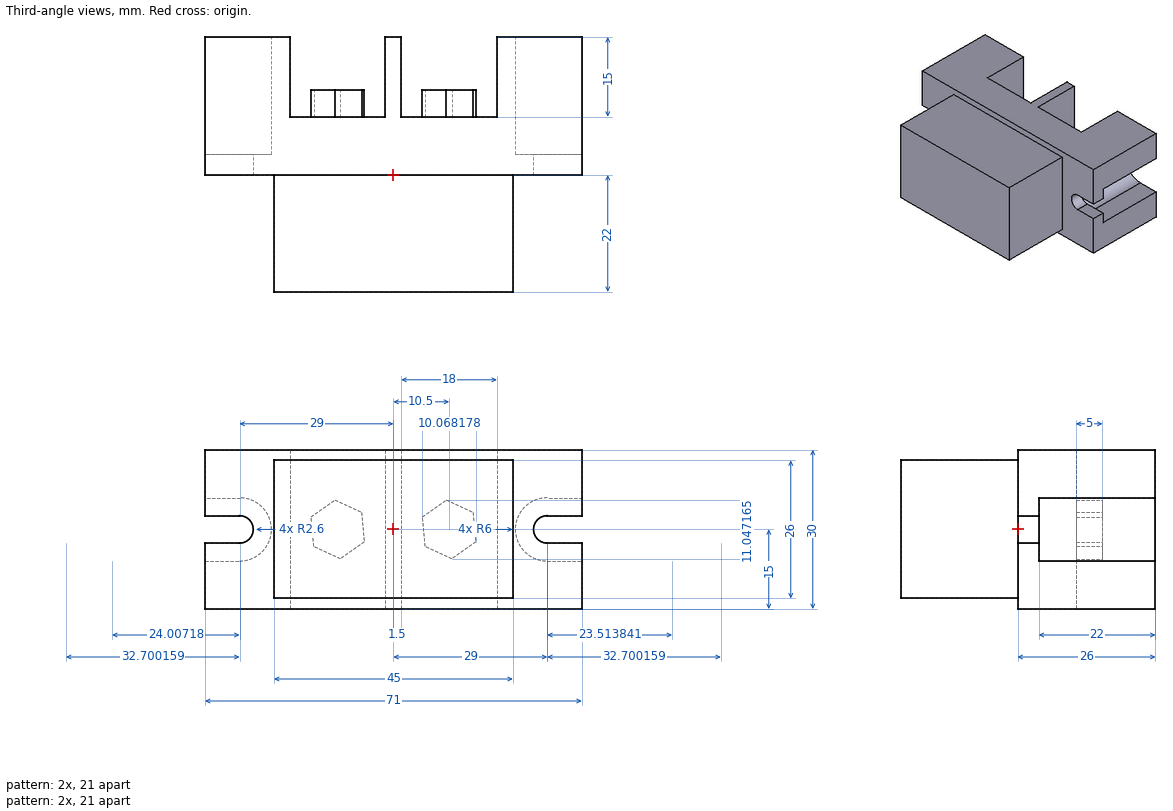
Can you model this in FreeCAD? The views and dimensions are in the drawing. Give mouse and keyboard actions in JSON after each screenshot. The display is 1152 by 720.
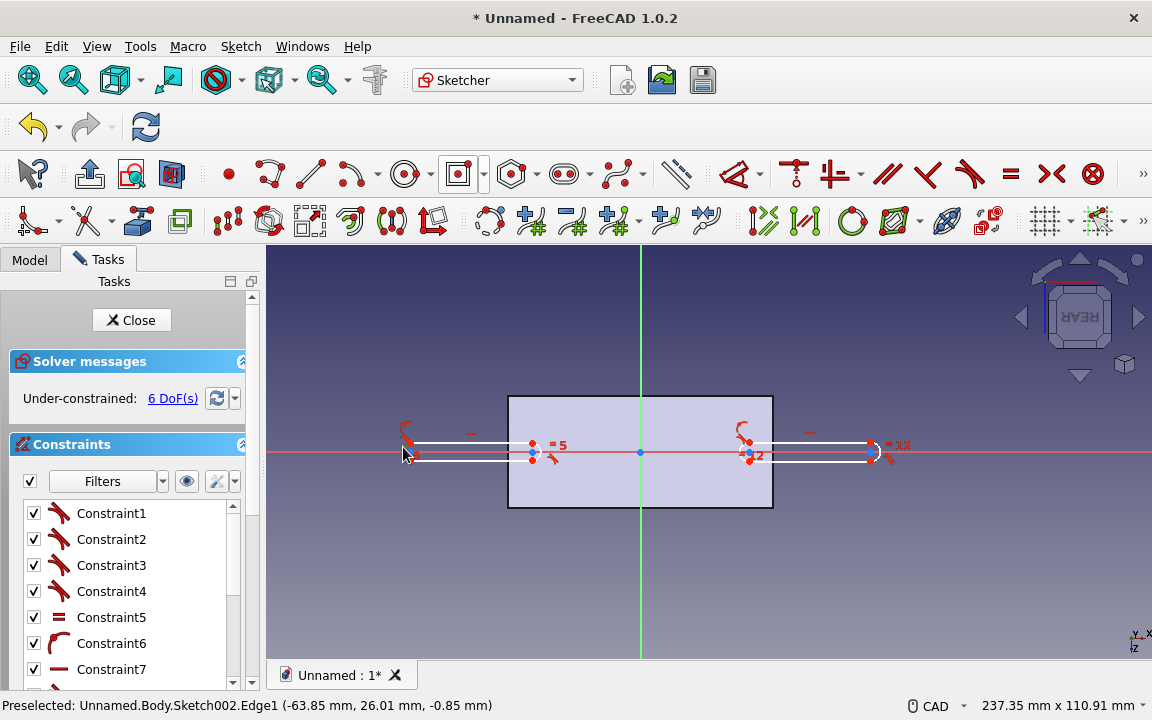
{"action": "scroll", "coordinate": [742, 447], "scroll_direction": "up", "scroll_amount": 5}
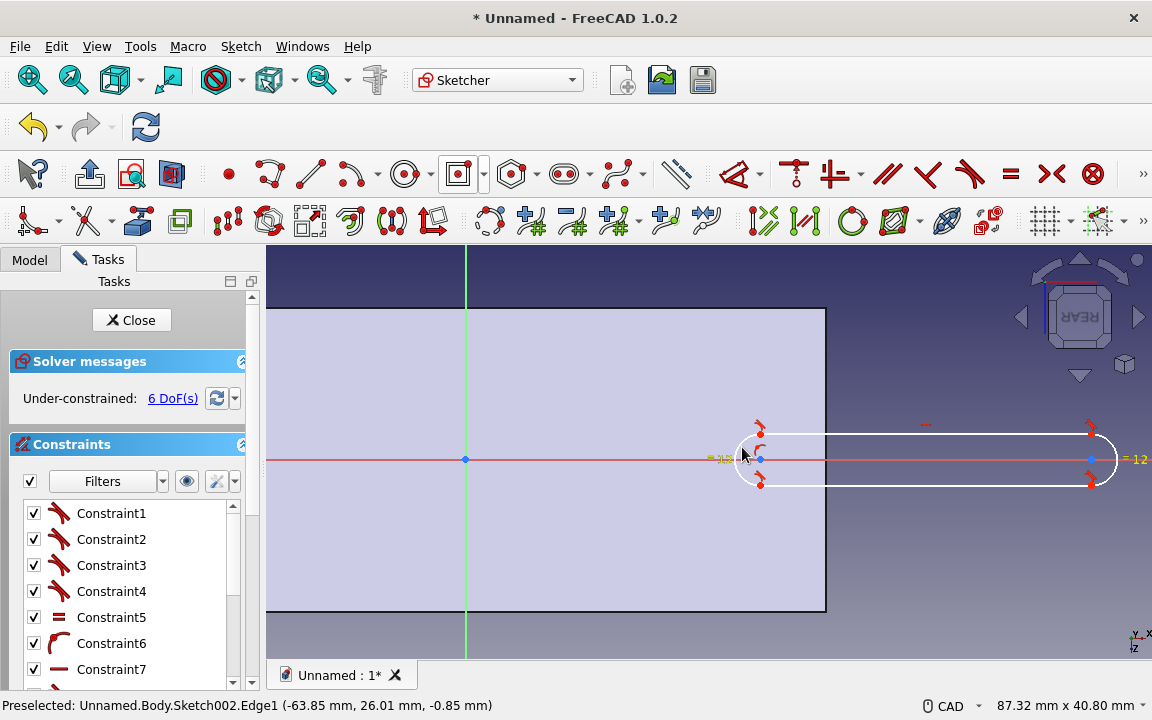
{"action": "left_click", "coordinate": [740, 445]}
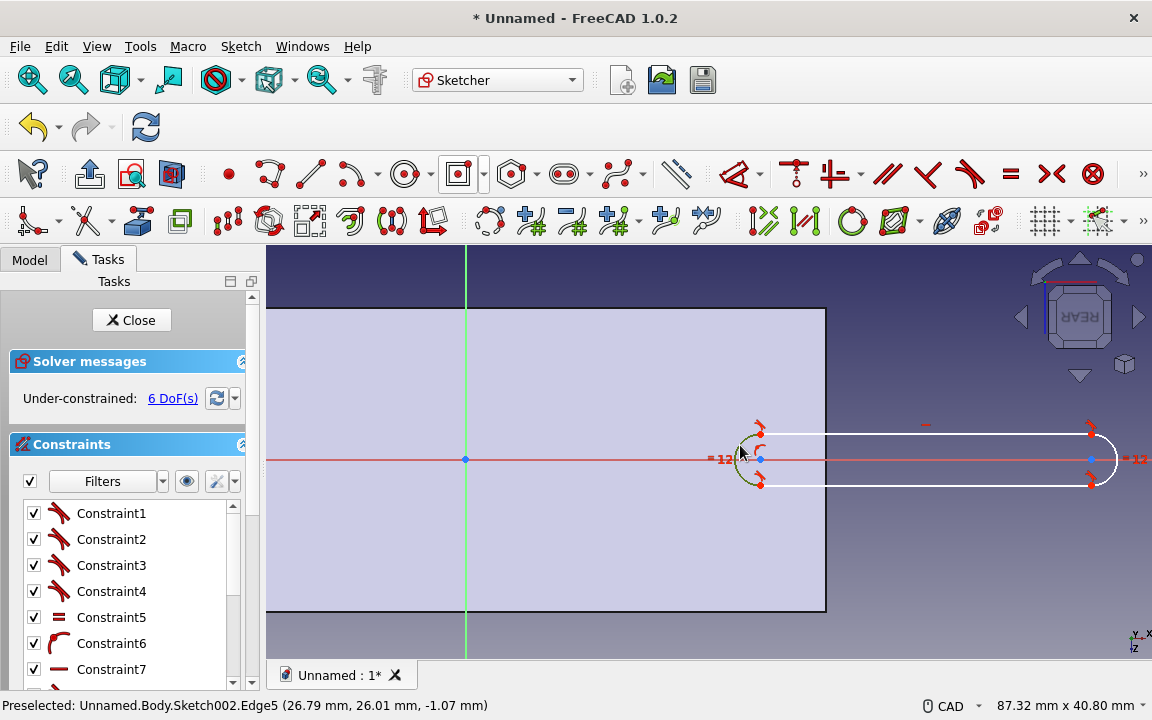
{"action": "left_click", "coordinate": [1011, 174]}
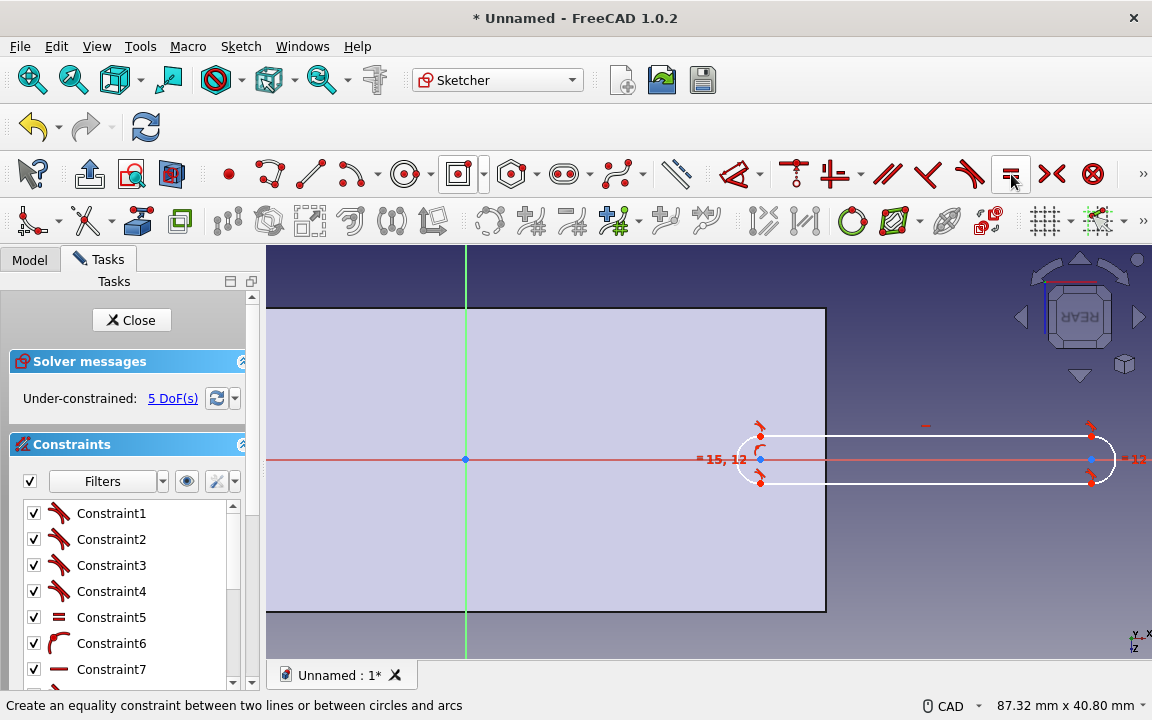
{"action": "scroll", "coordinate": [742, 447], "scroll_direction": "down", "scroll_amount": 5}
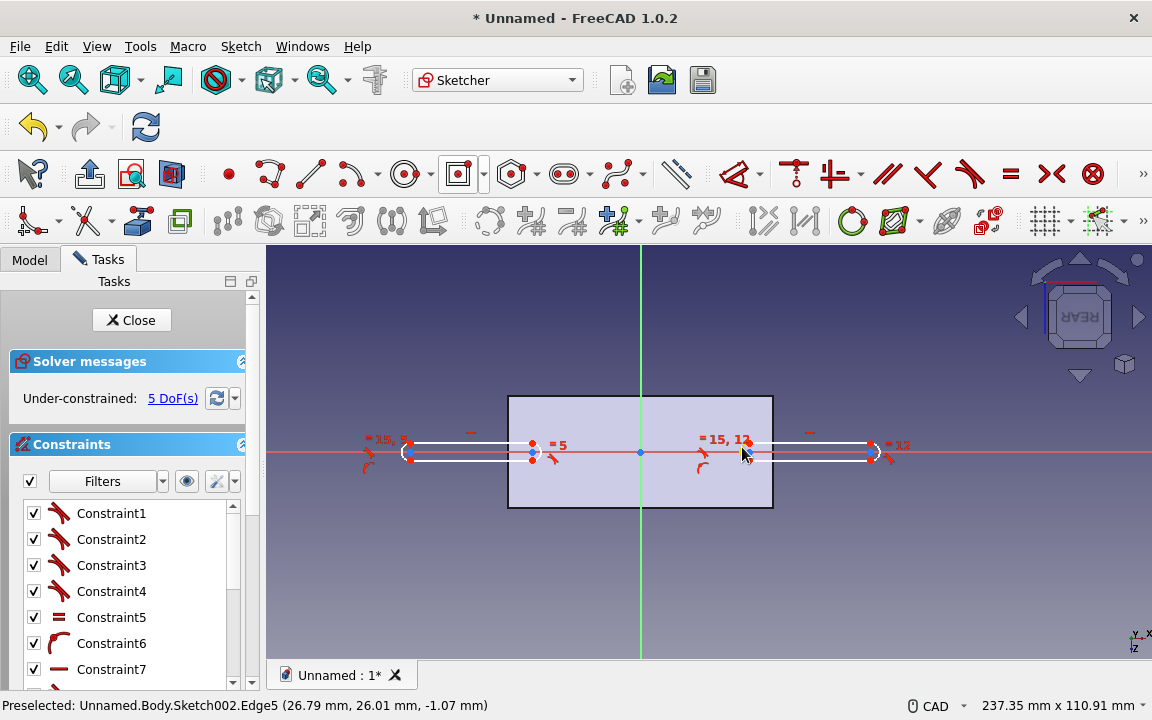
{"action": "scroll", "coordinate": [403, 447], "scroll_direction": "up", "scroll_amount": 8}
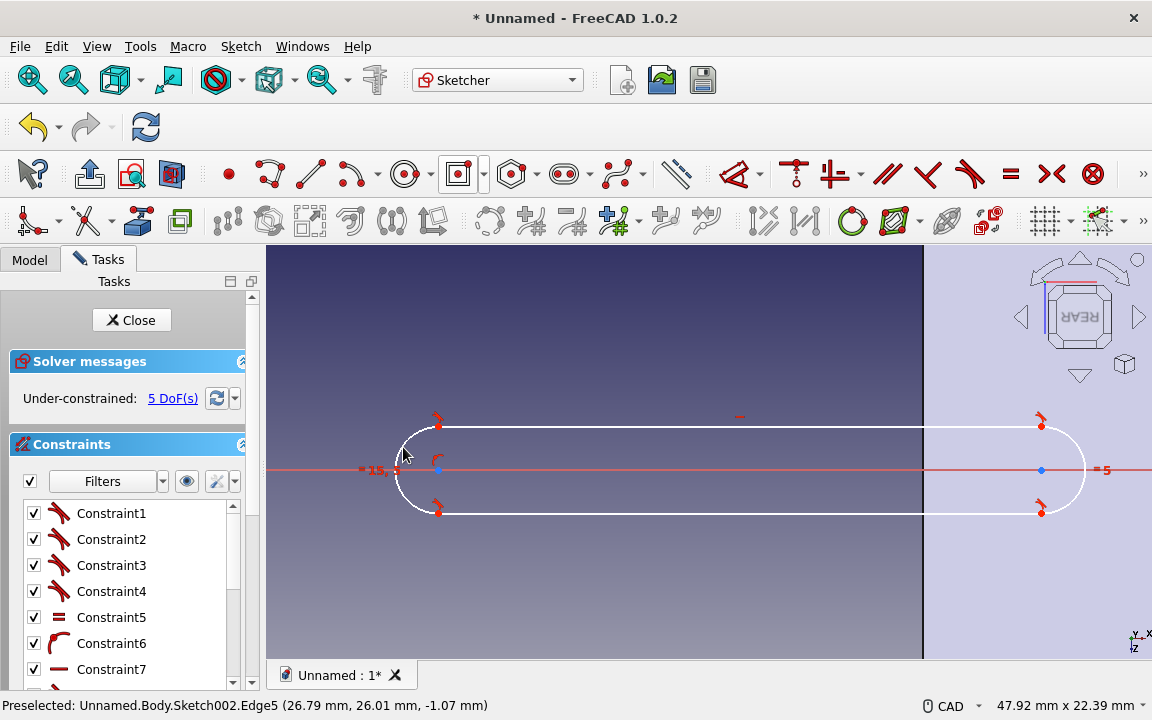
{"action": "left_click", "coordinate": [404, 445]}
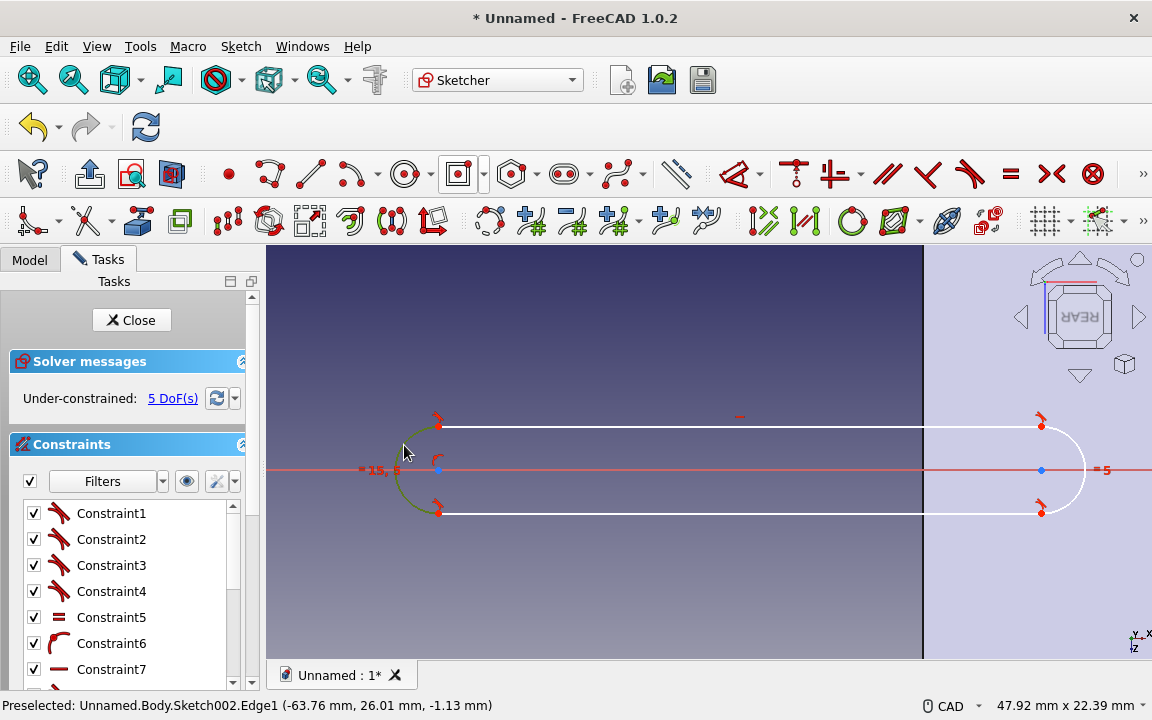
{"action": "left_click", "coordinate": [760, 174]}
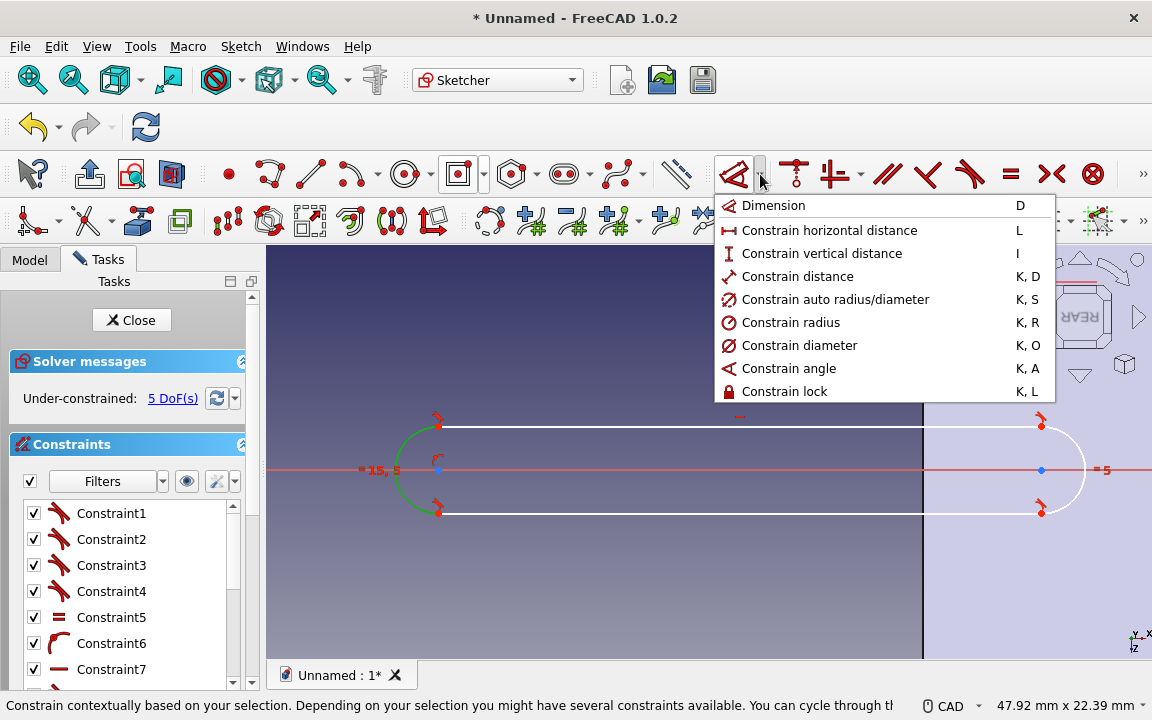
{"action": "left_click", "coordinate": [885, 322]}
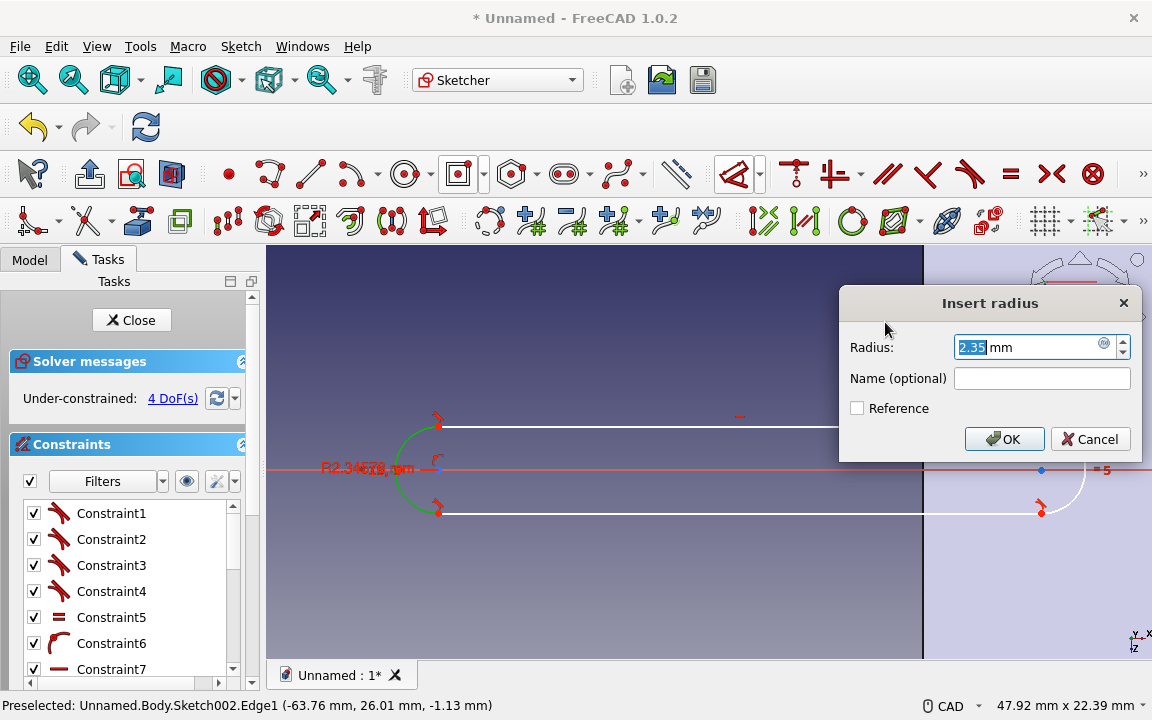
{"action": "type", "text": "2.6"}
{"action": "key", "text": "Return"}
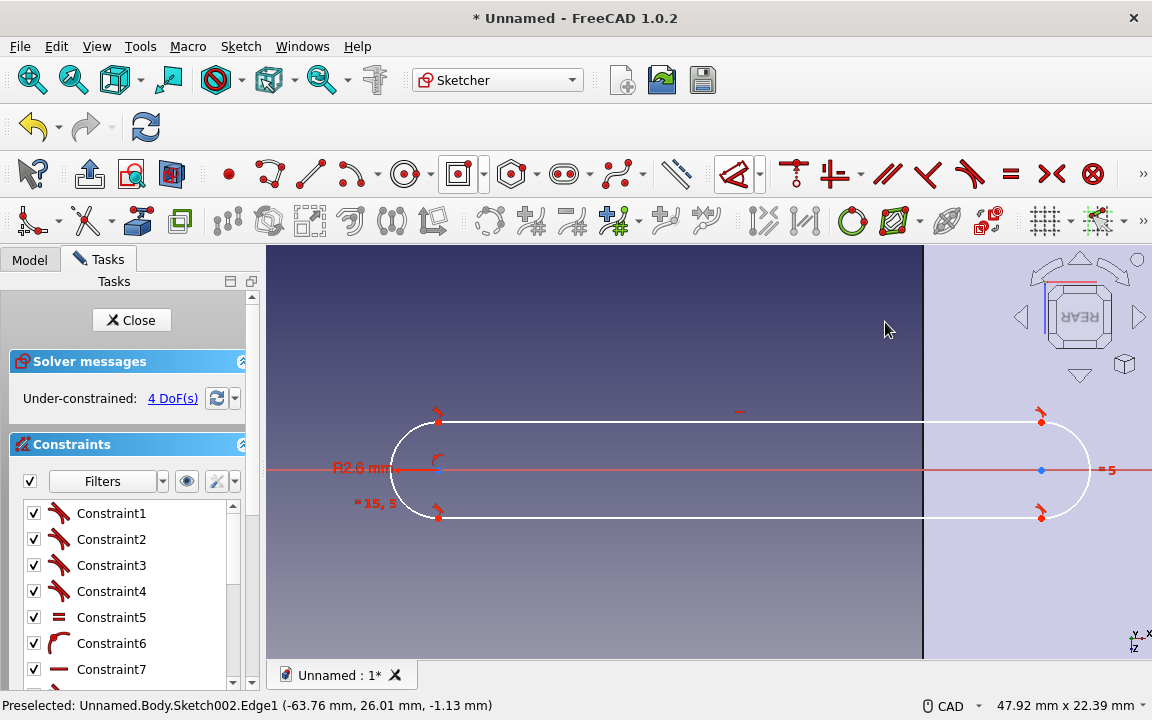
{"action": "scroll", "coordinate": [403, 447], "scroll_direction": "down", "scroll_amount": 8}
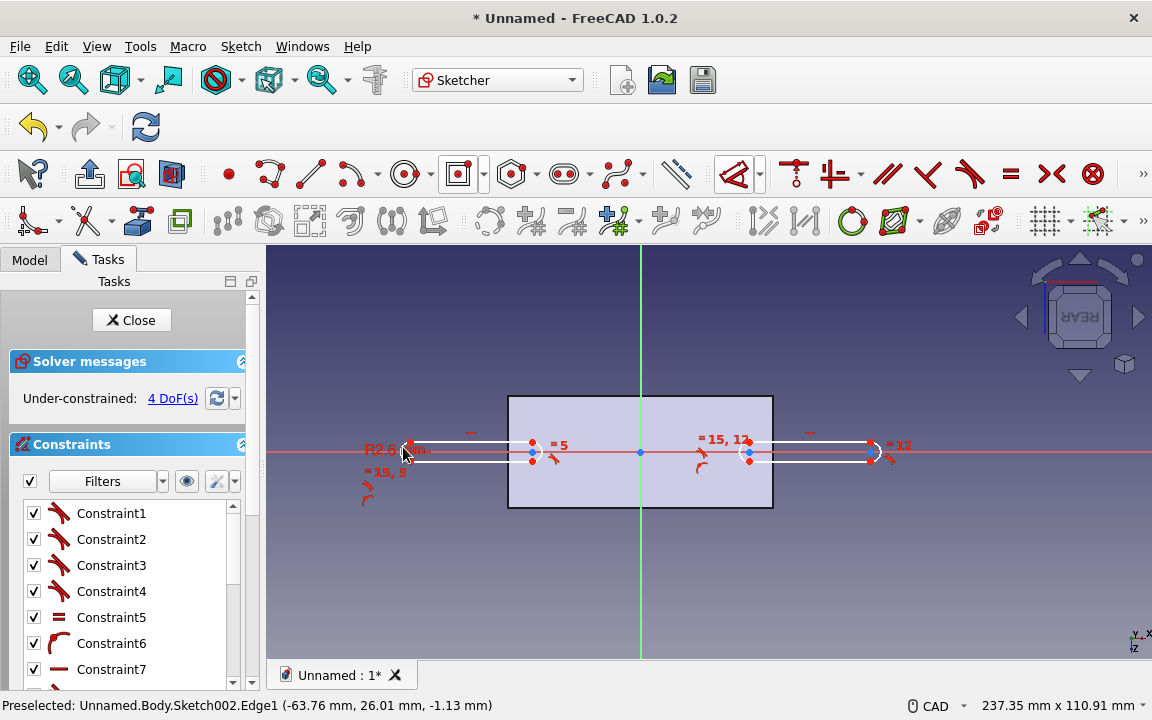
{"action": "scroll", "coordinate": [532, 462], "scroll_direction": "up", "scroll_amount": 2}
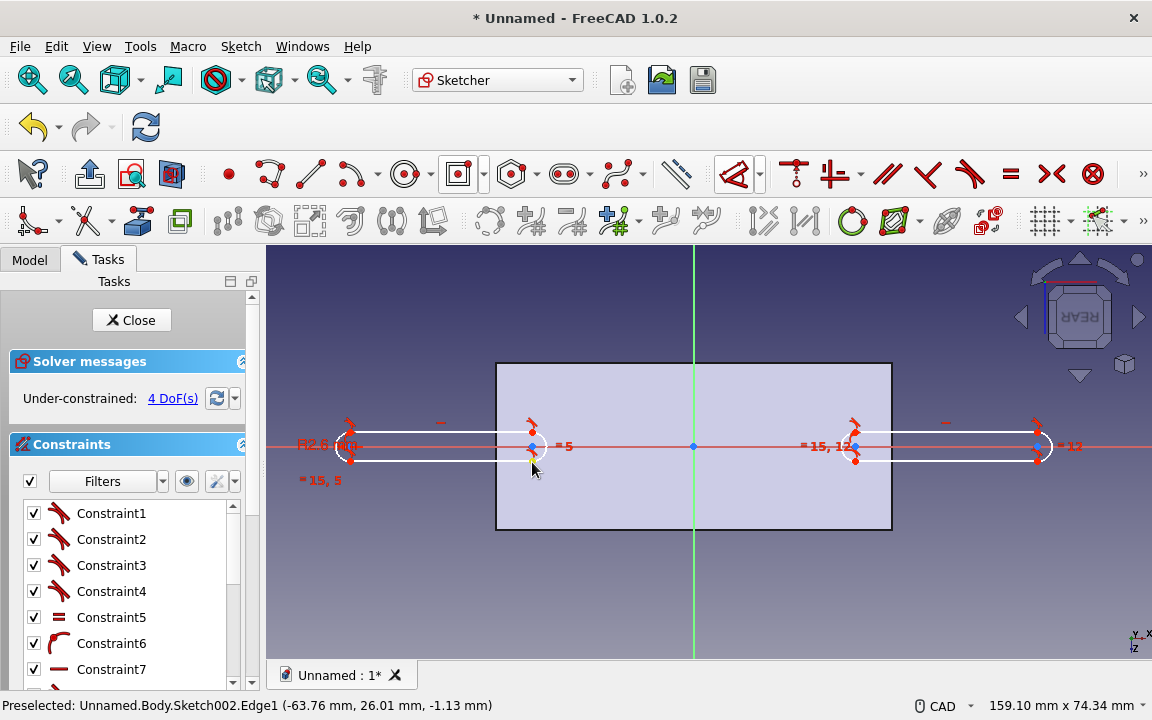
{"action": "left_click", "coordinate": [532, 461]}